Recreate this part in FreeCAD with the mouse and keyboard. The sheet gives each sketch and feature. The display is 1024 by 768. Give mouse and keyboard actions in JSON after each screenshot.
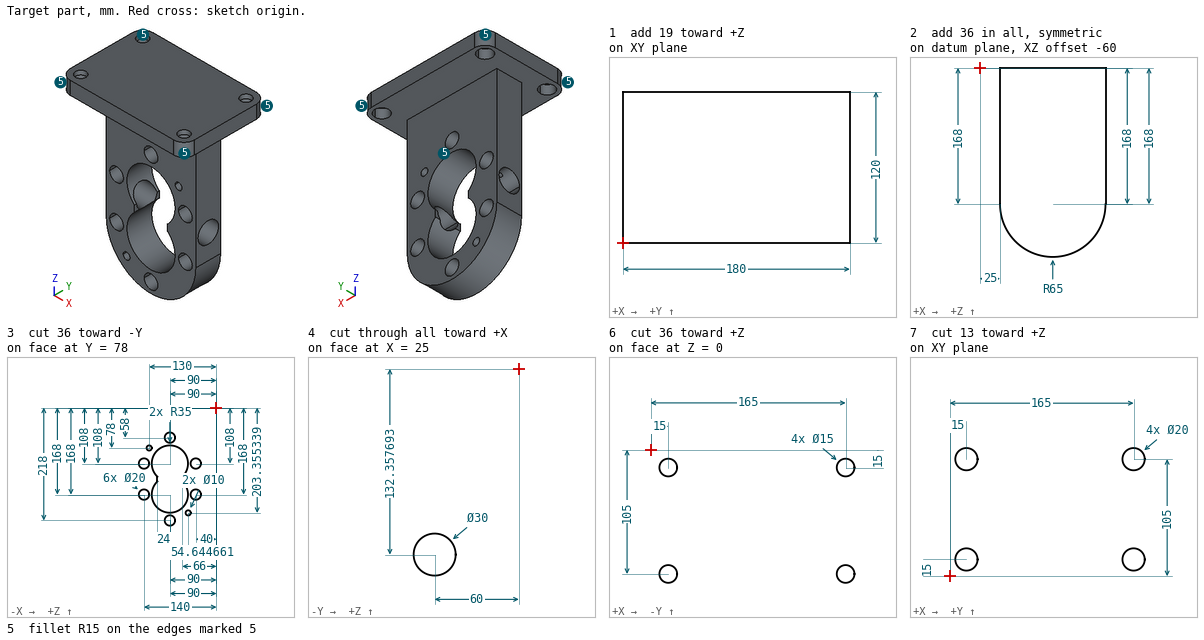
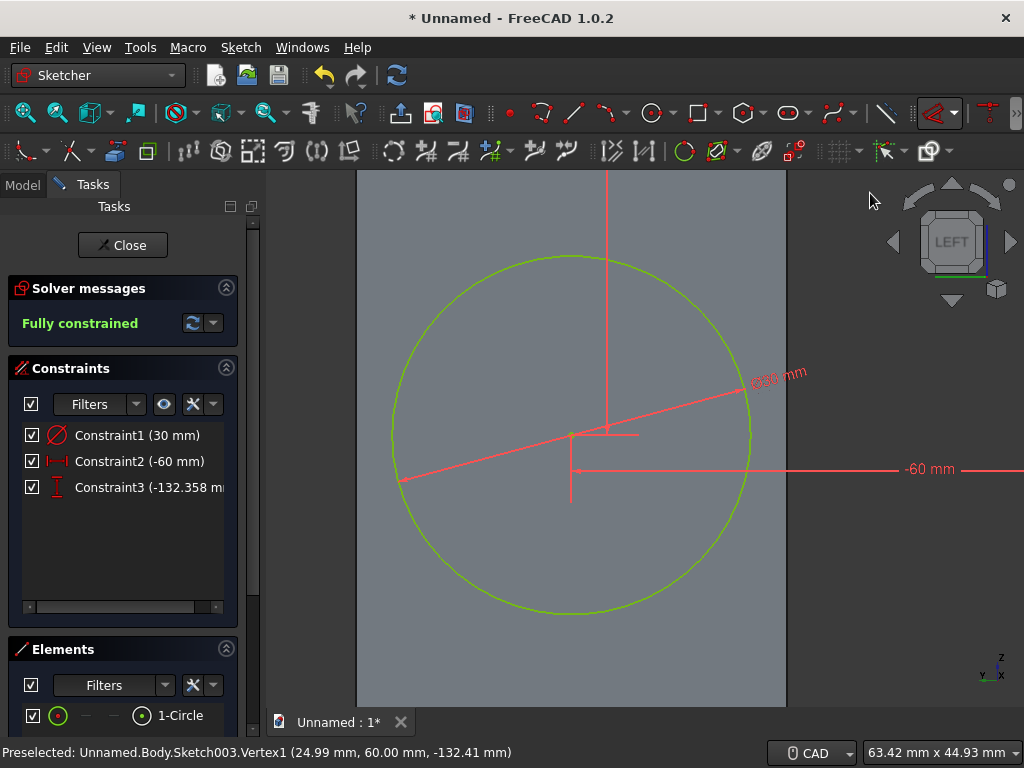
{"action": "left_click", "coordinate": [123, 245]}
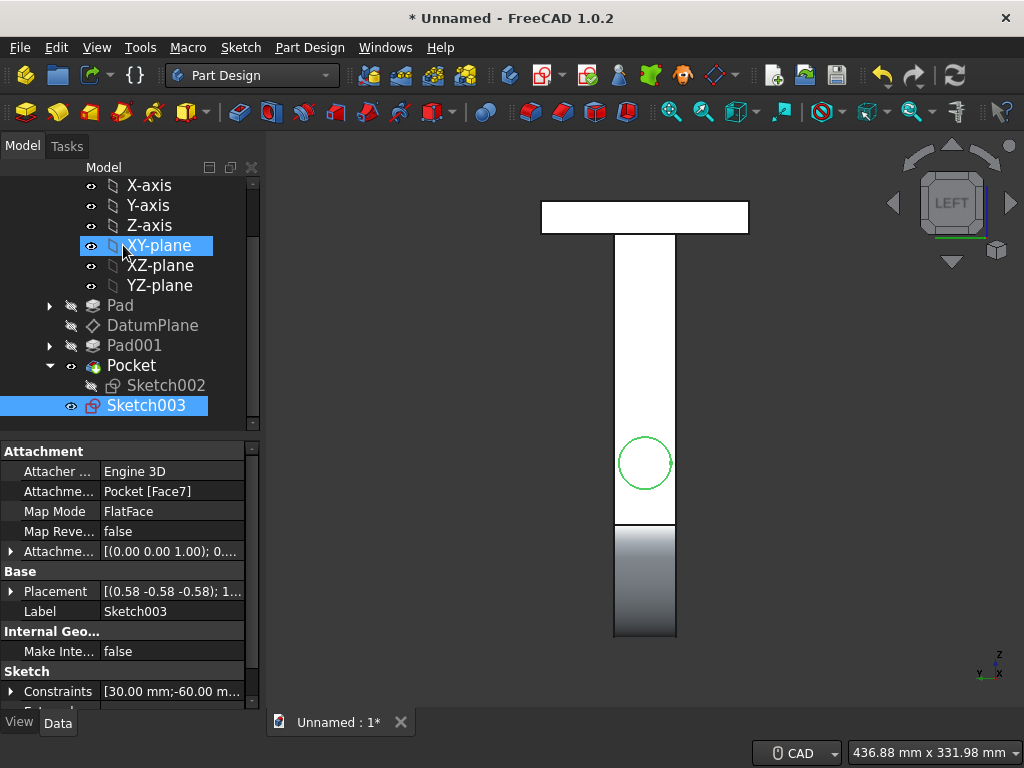
{"action": "left_click", "coordinate": [240, 112]}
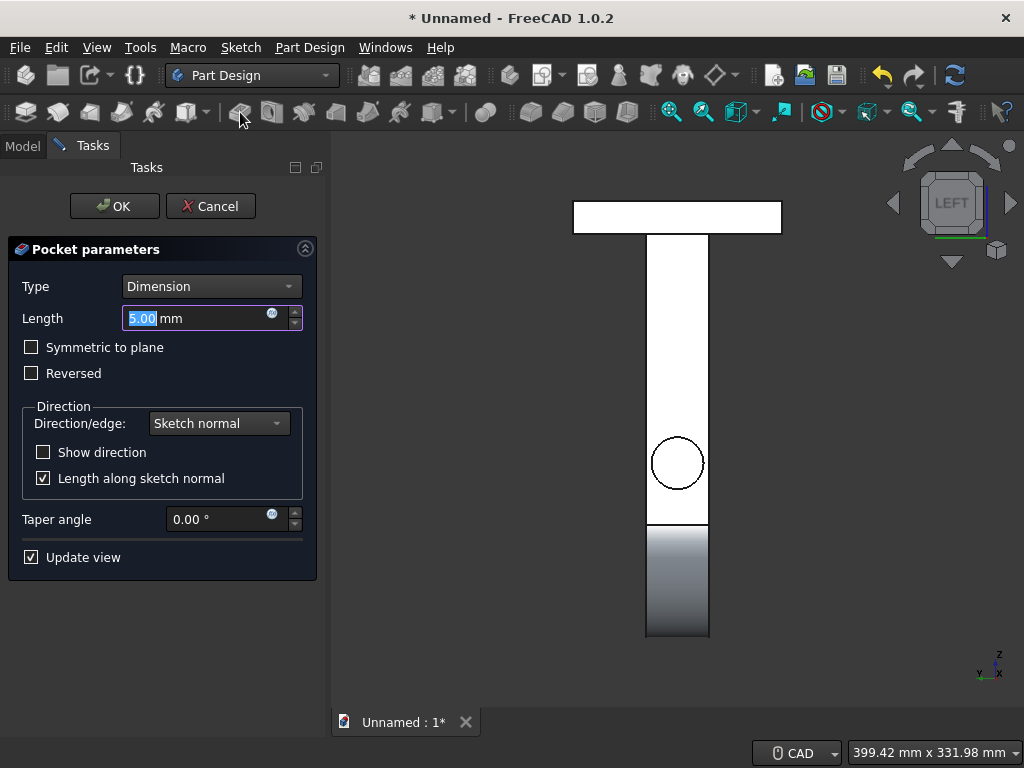
{"action": "left_click", "coordinate": [212, 286]}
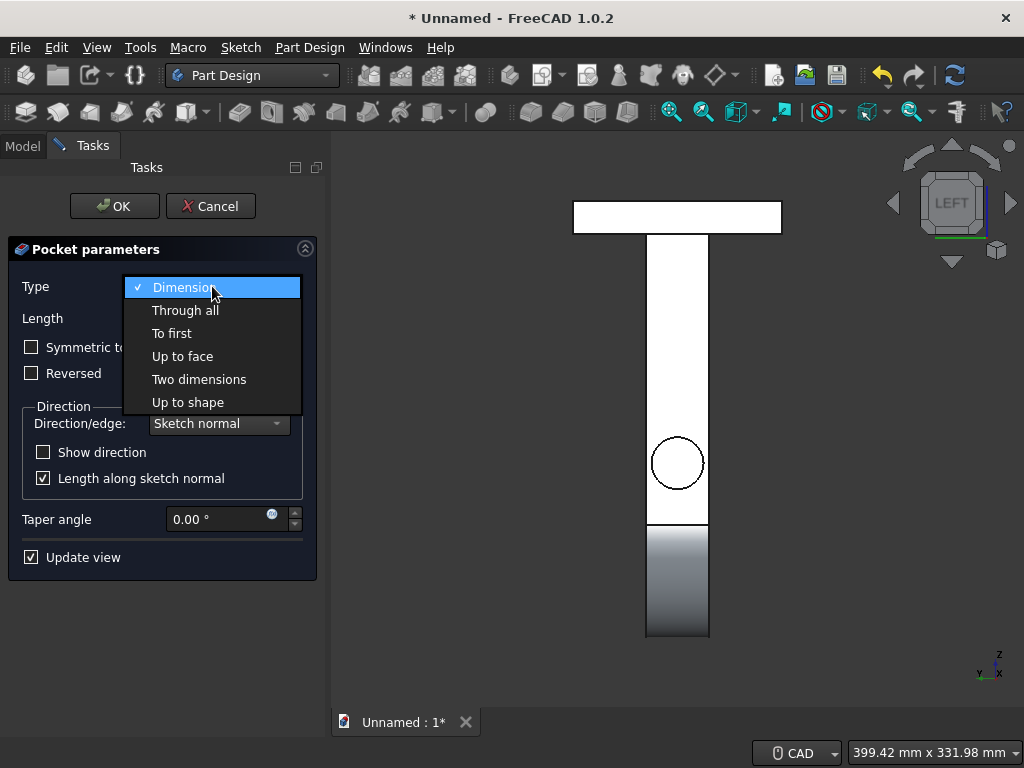
{"action": "left_click", "coordinate": [212, 310]}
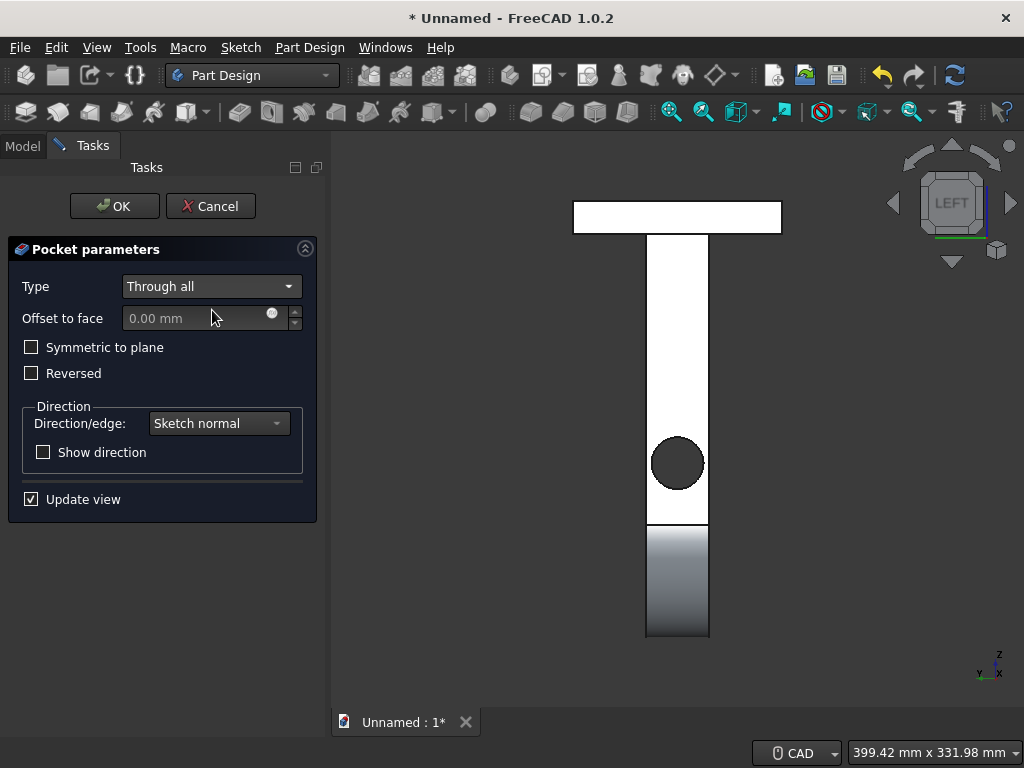
{"action": "left_click", "coordinate": [115, 206]}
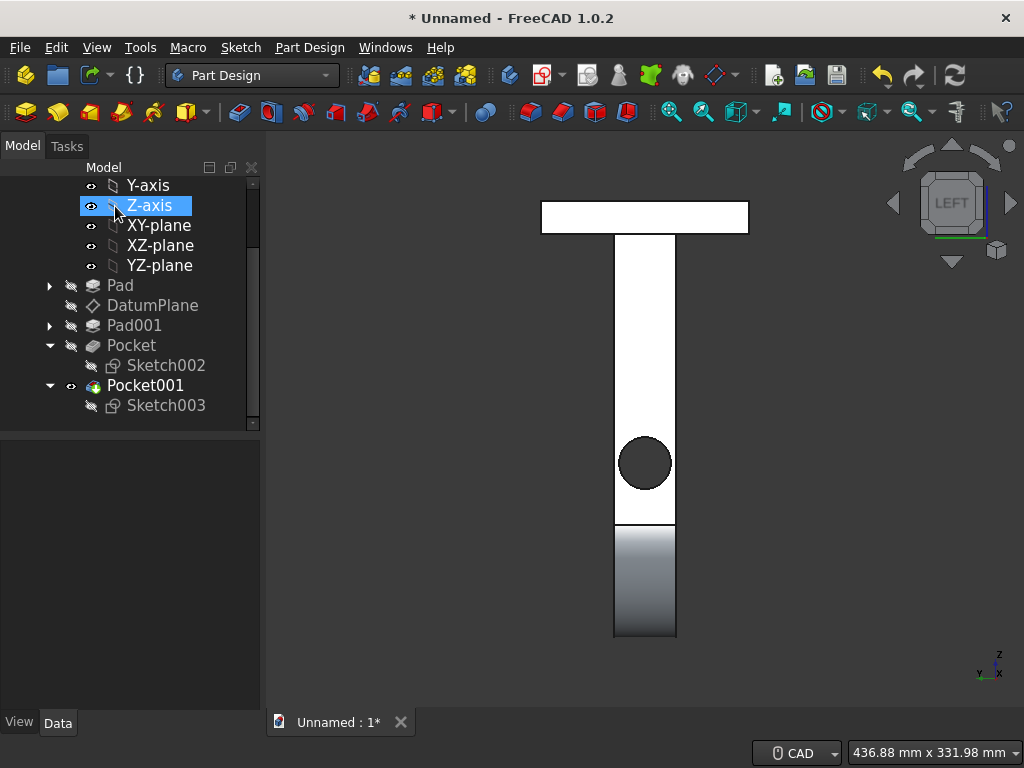
{"action": "left_click", "coordinate": [541, 216]}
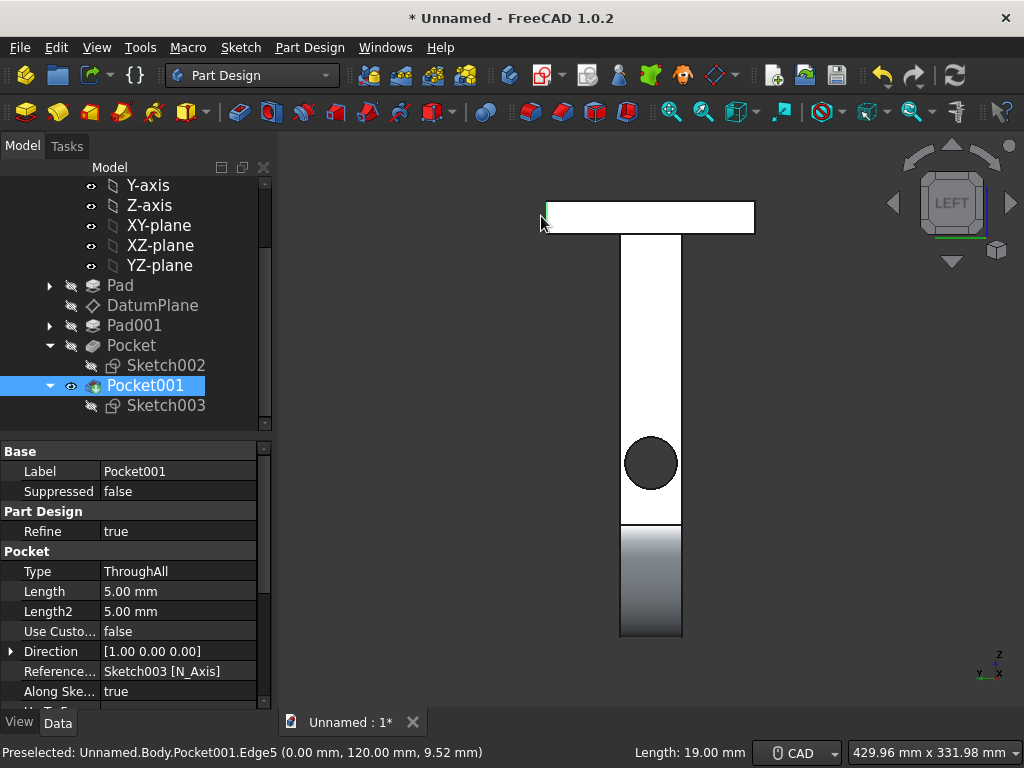
{"action": "left_click", "coordinate": [755, 216], "text": "ctrl"}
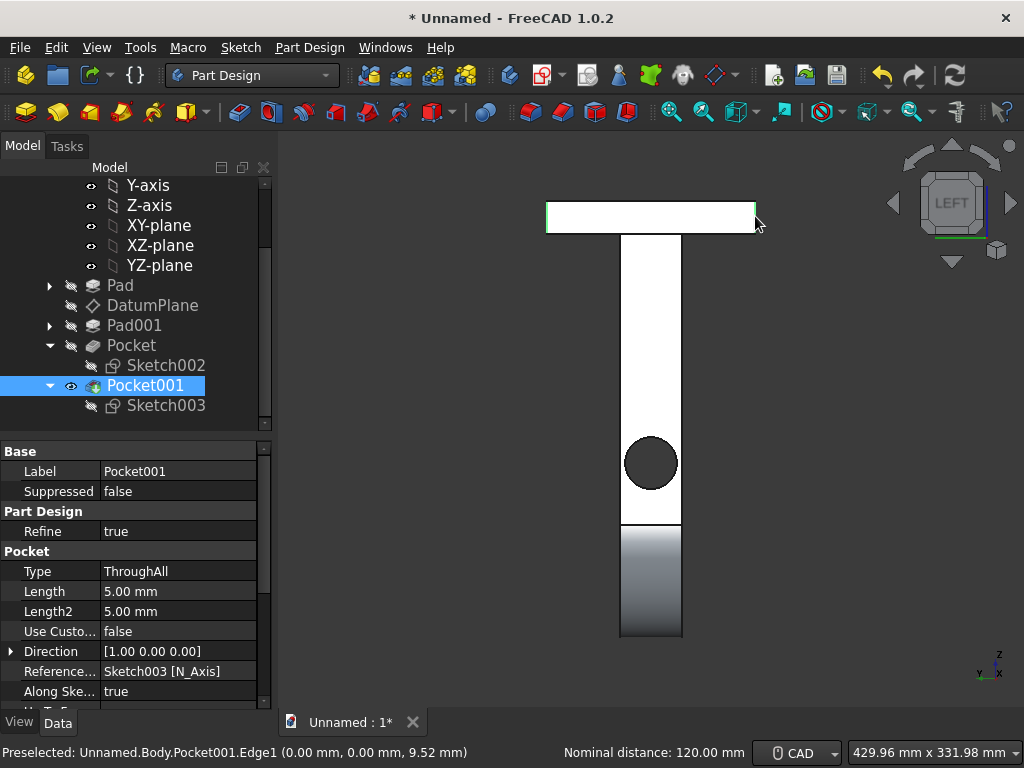
{"action": "key", "text": "0"}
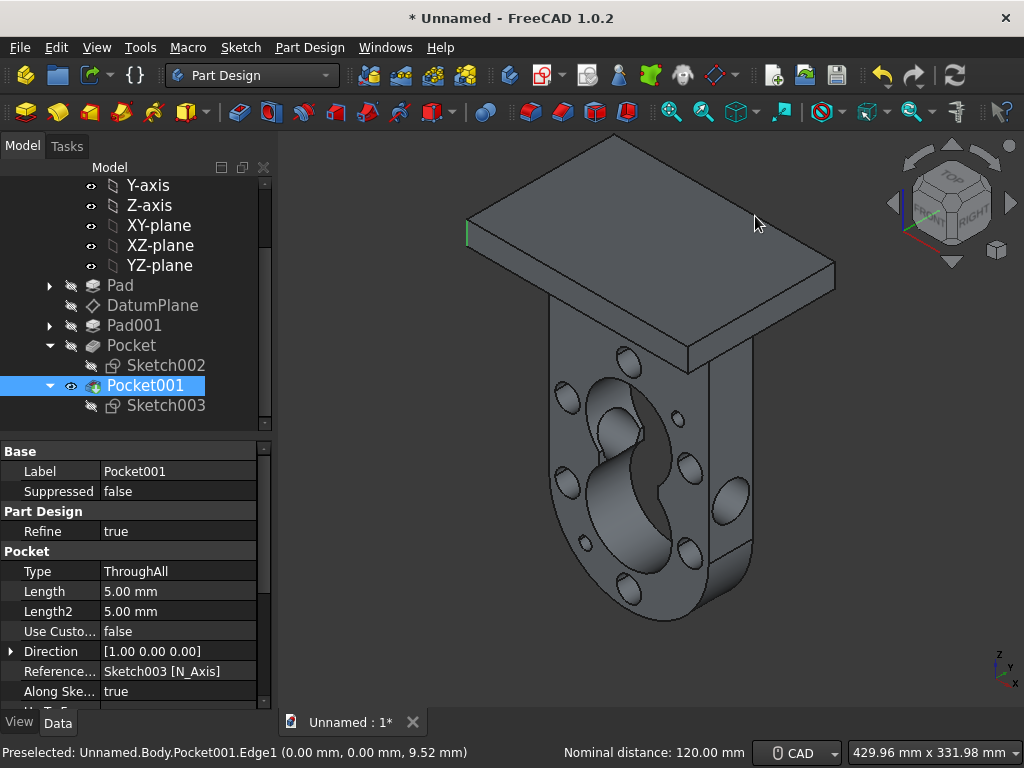
{"action": "left_click", "coordinate": [688, 359], "text": "ctrl"}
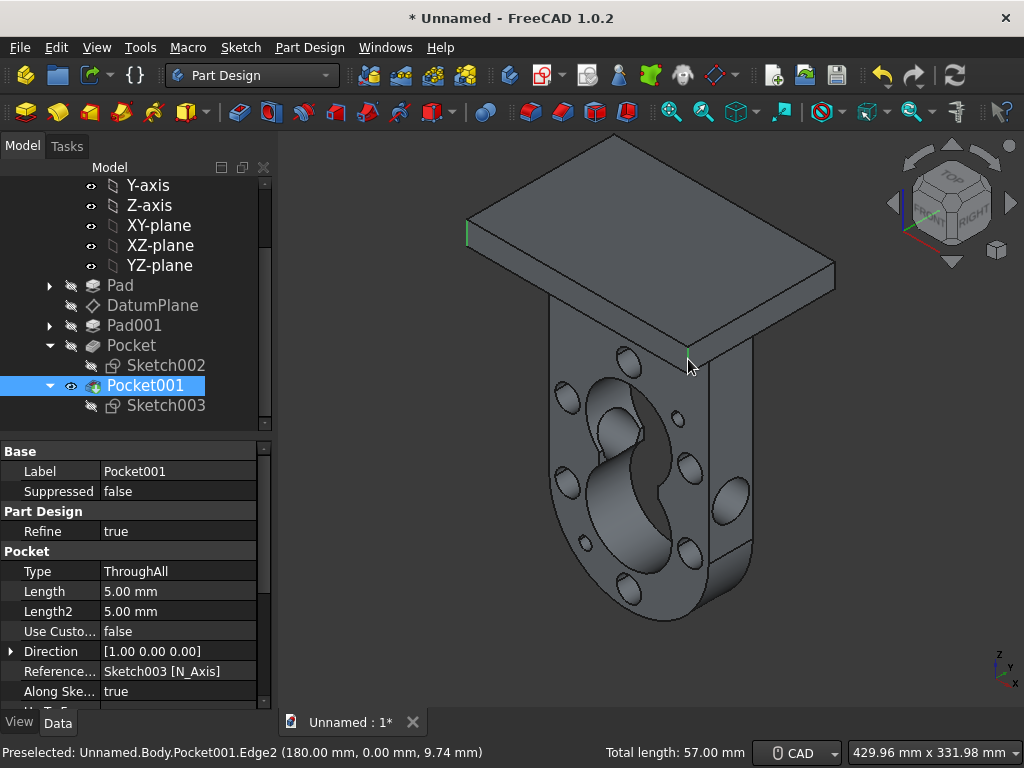
{"action": "key", "text": "2"}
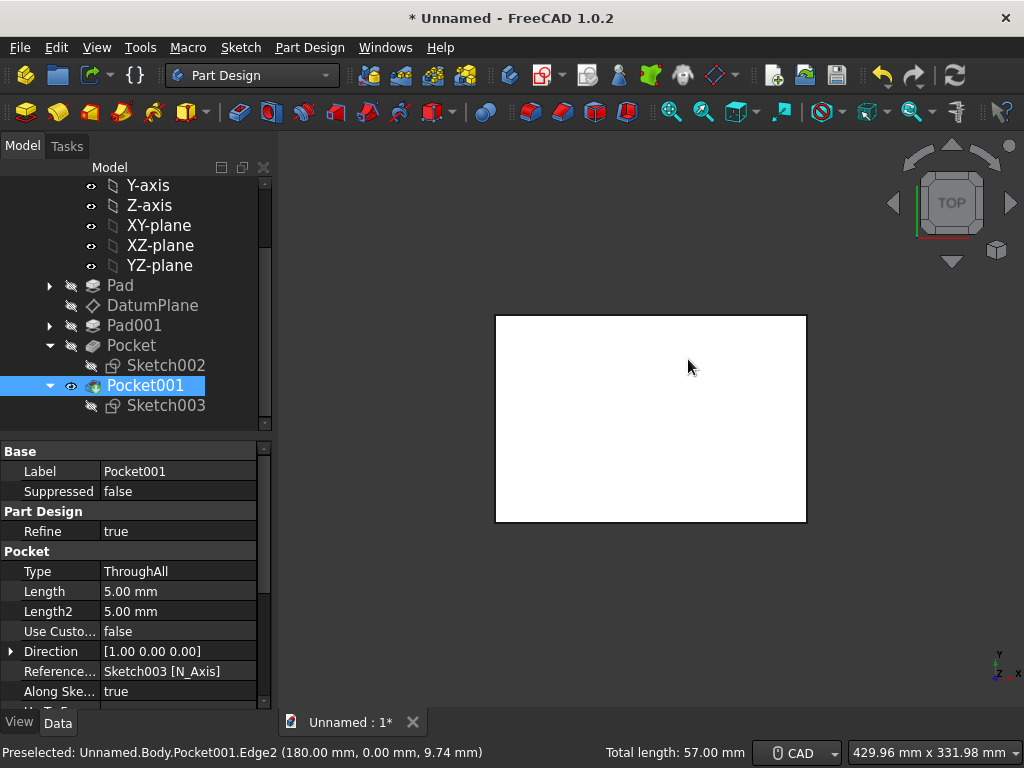
{"action": "left_click", "coordinate": [672, 112]}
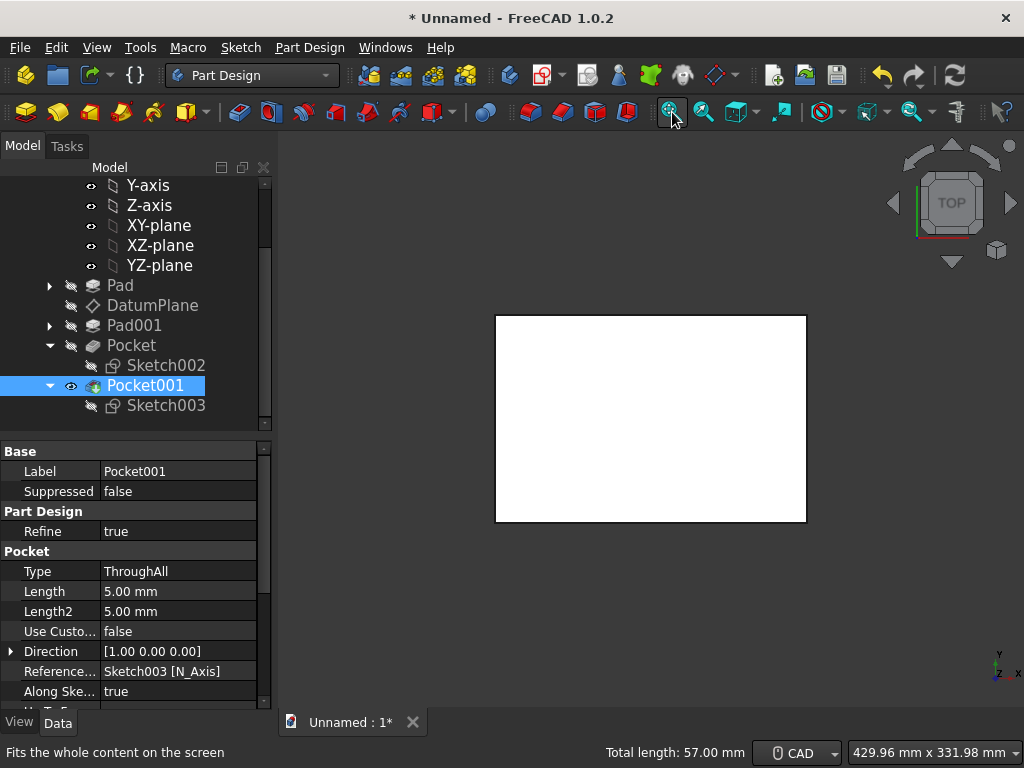
{"action": "key", "text": "1"}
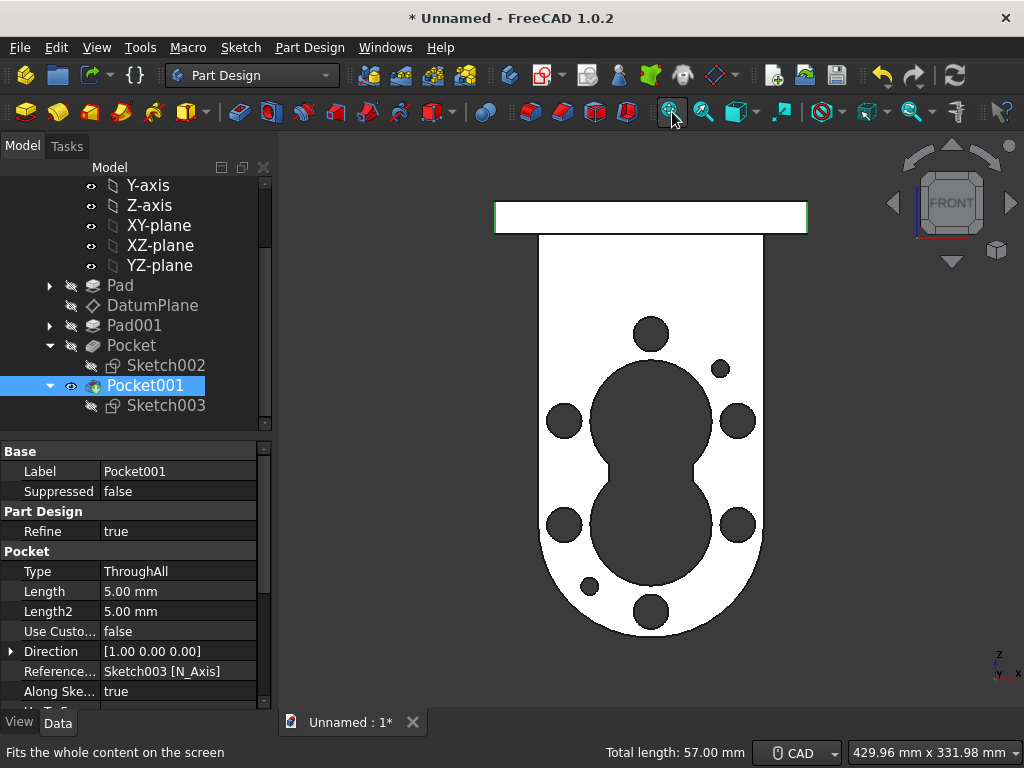
{"action": "key", "text": "3"}